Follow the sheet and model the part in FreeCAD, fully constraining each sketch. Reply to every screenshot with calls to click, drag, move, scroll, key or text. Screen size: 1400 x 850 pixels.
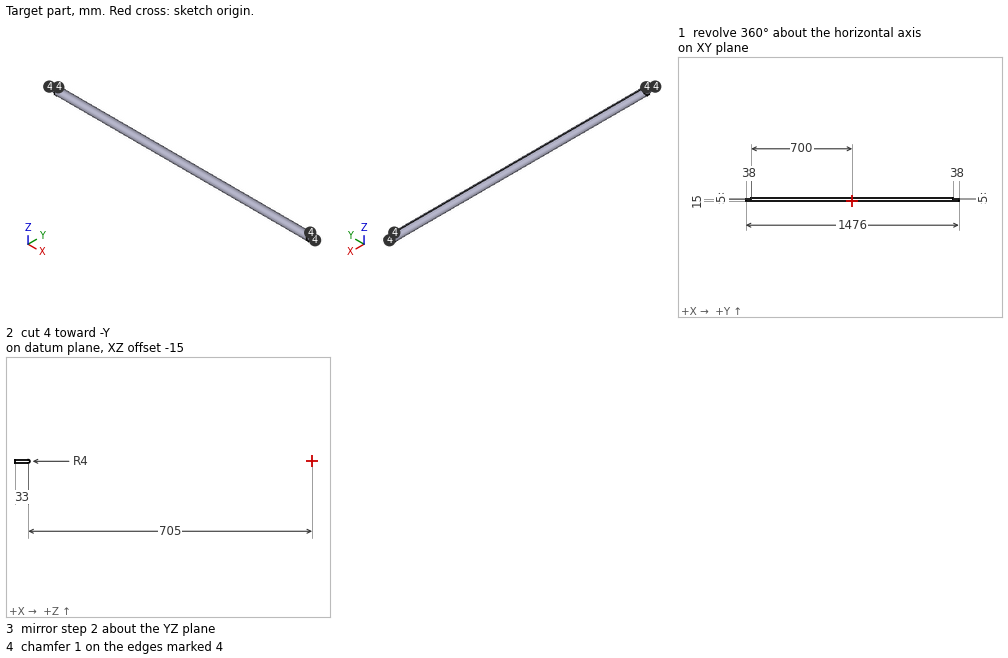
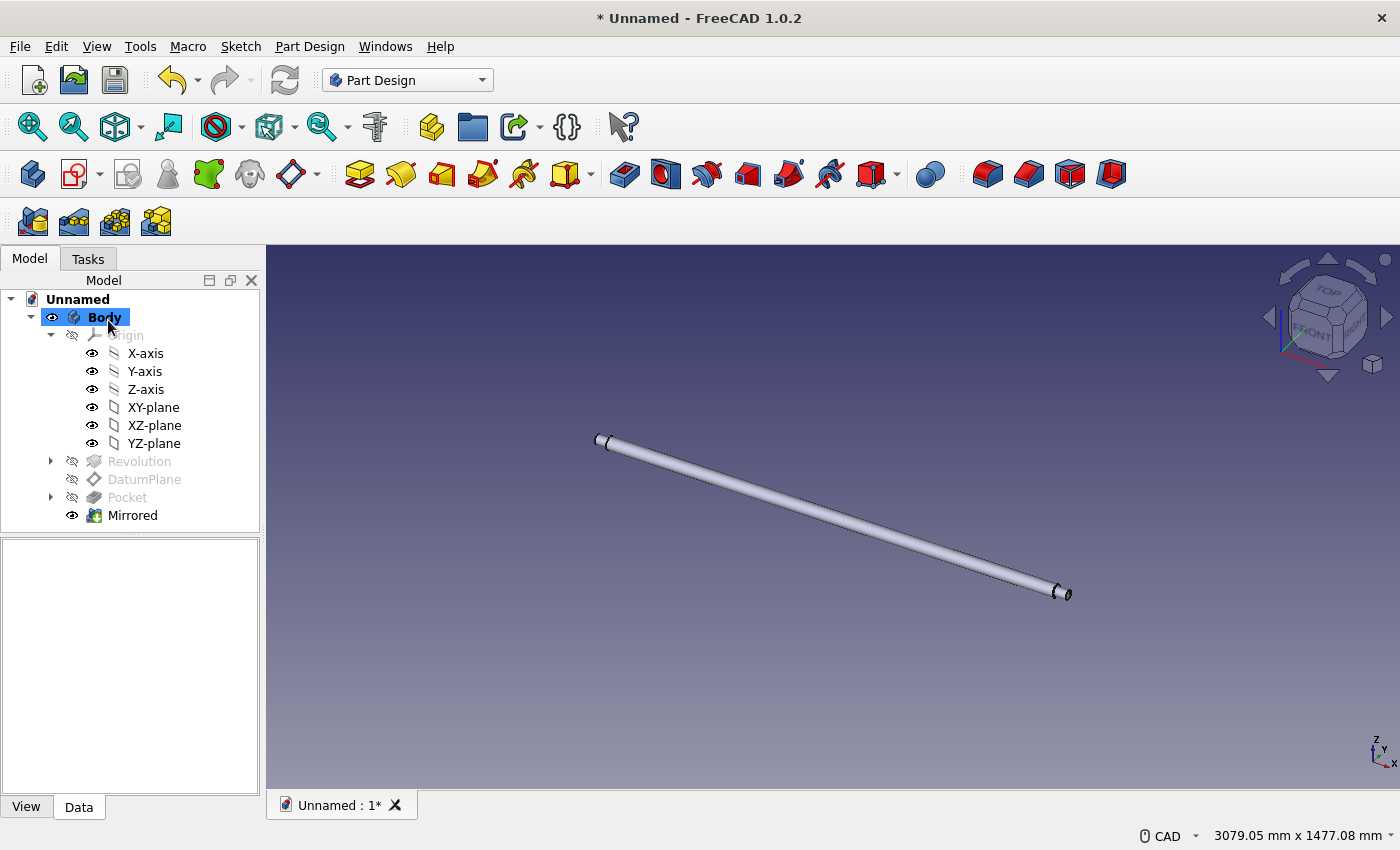
click(33, 128)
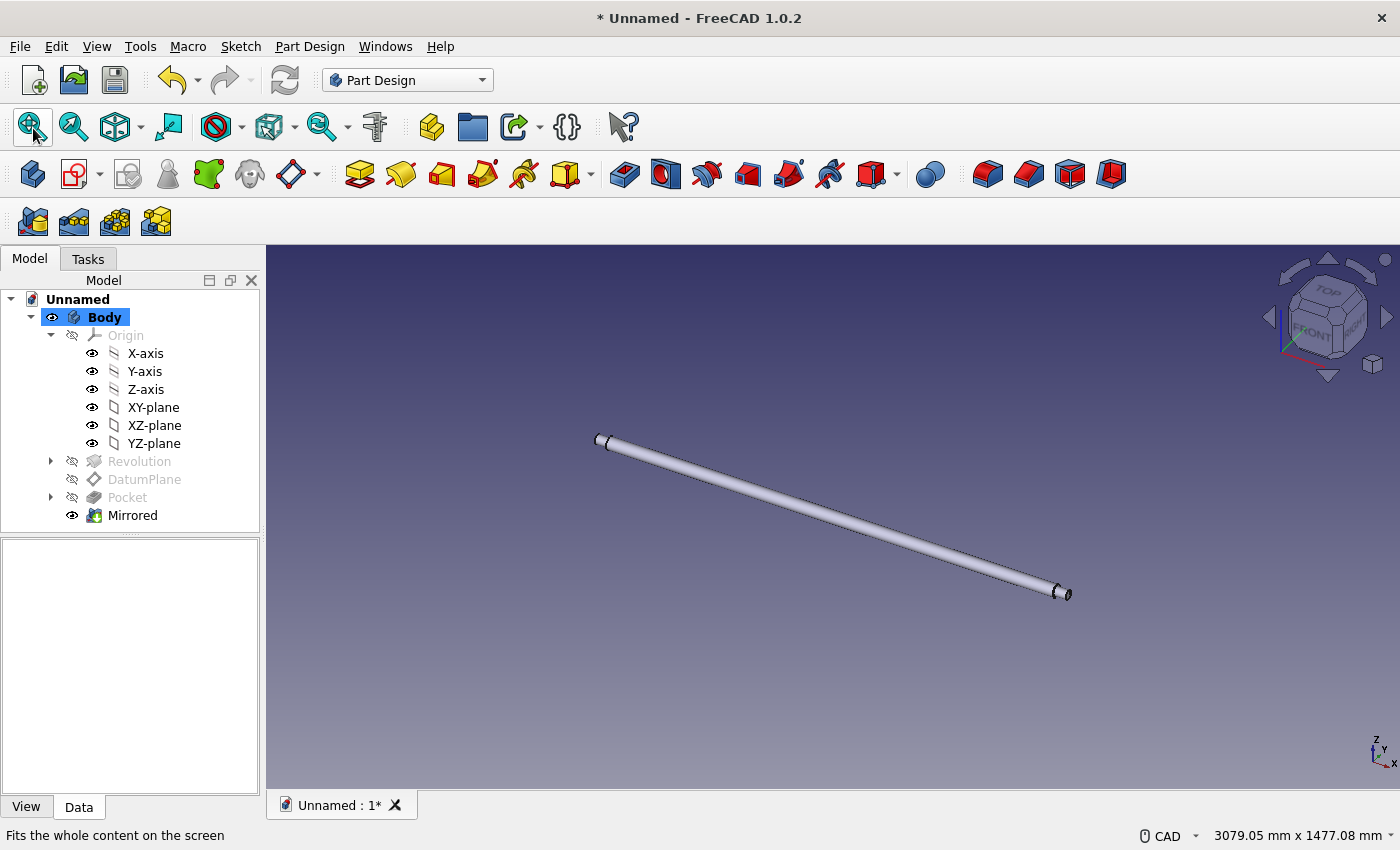
click(595, 441)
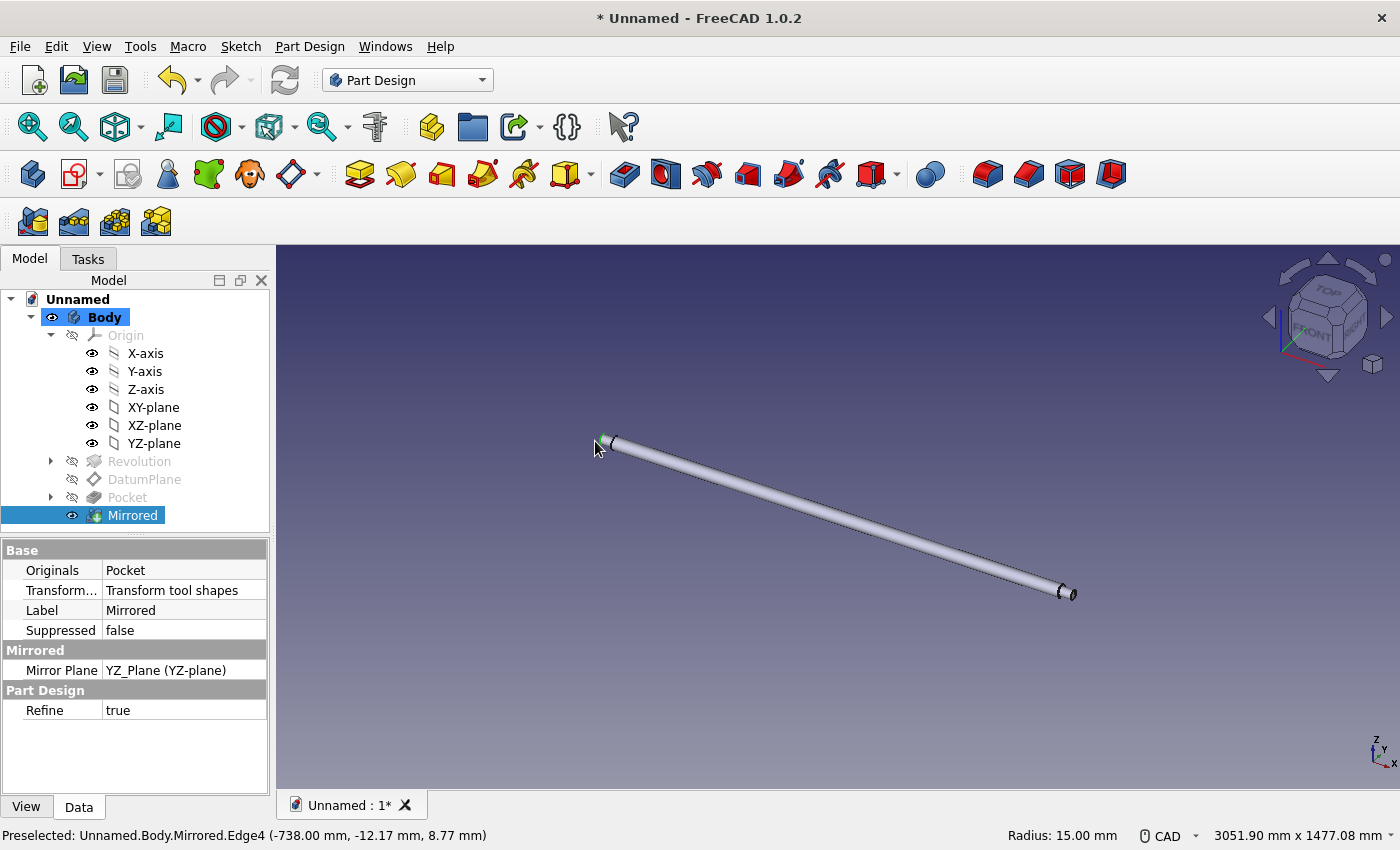
click(1071, 597, ctrl)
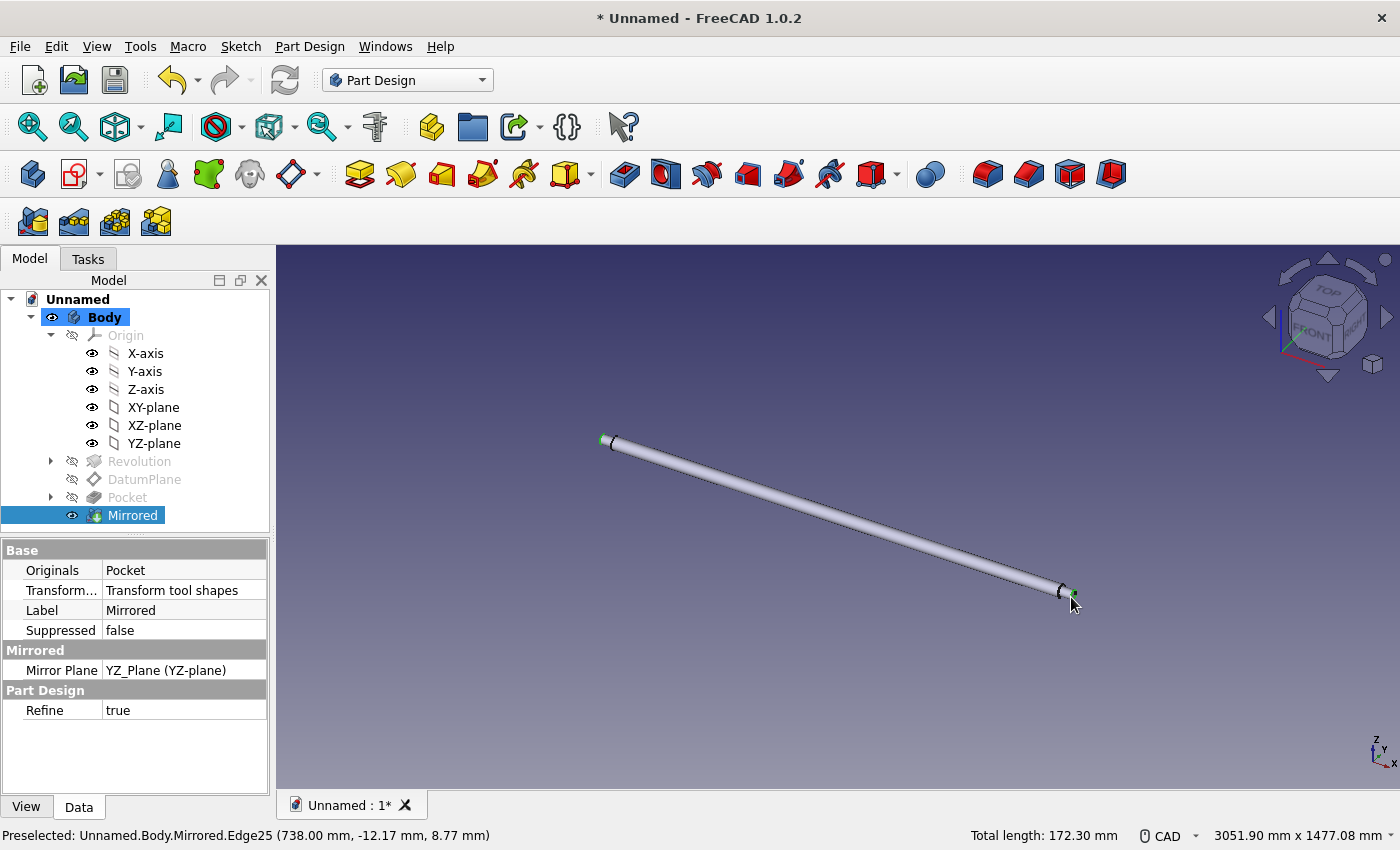
click(1058, 594, ctrl)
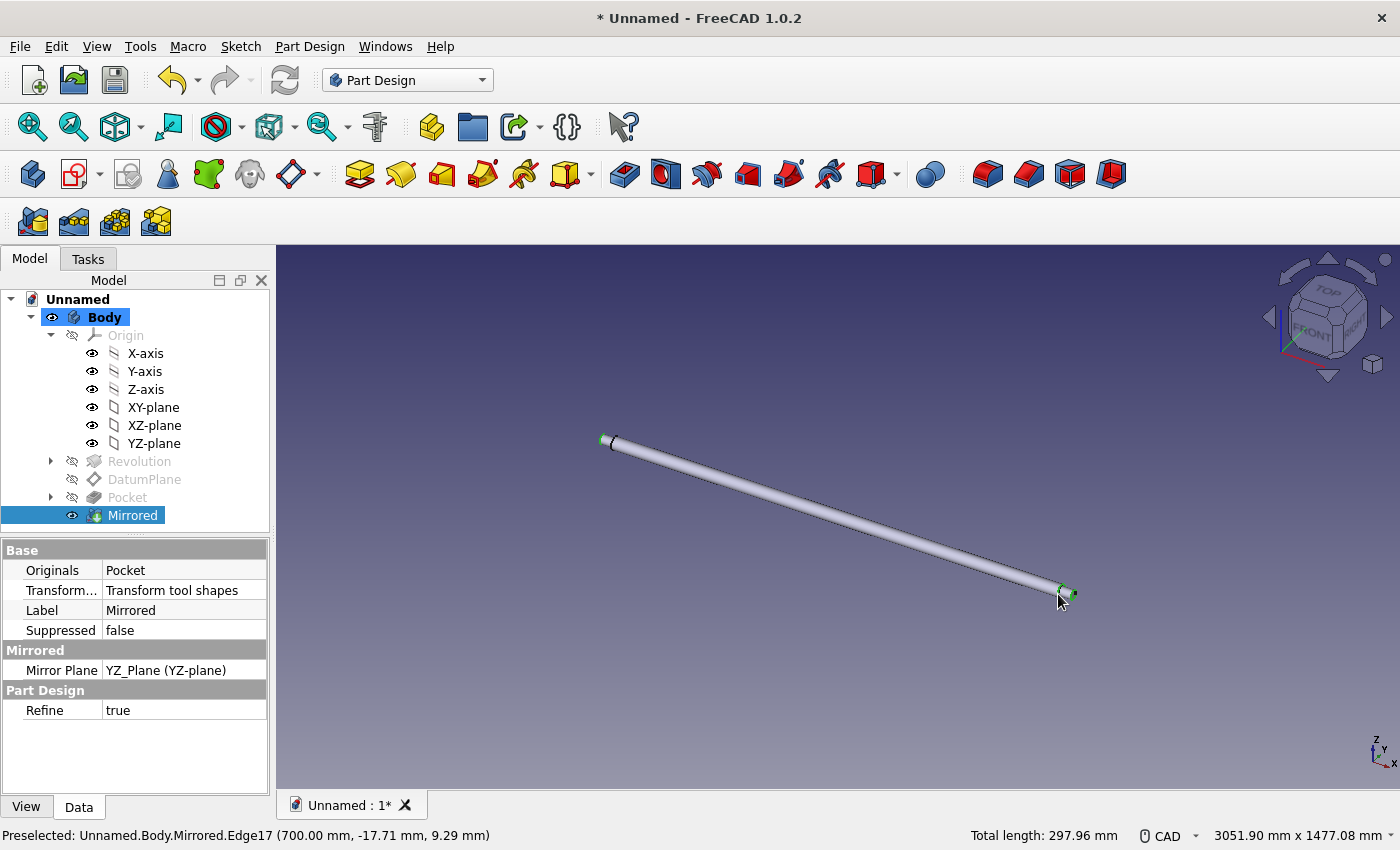
click(611, 446, ctrl)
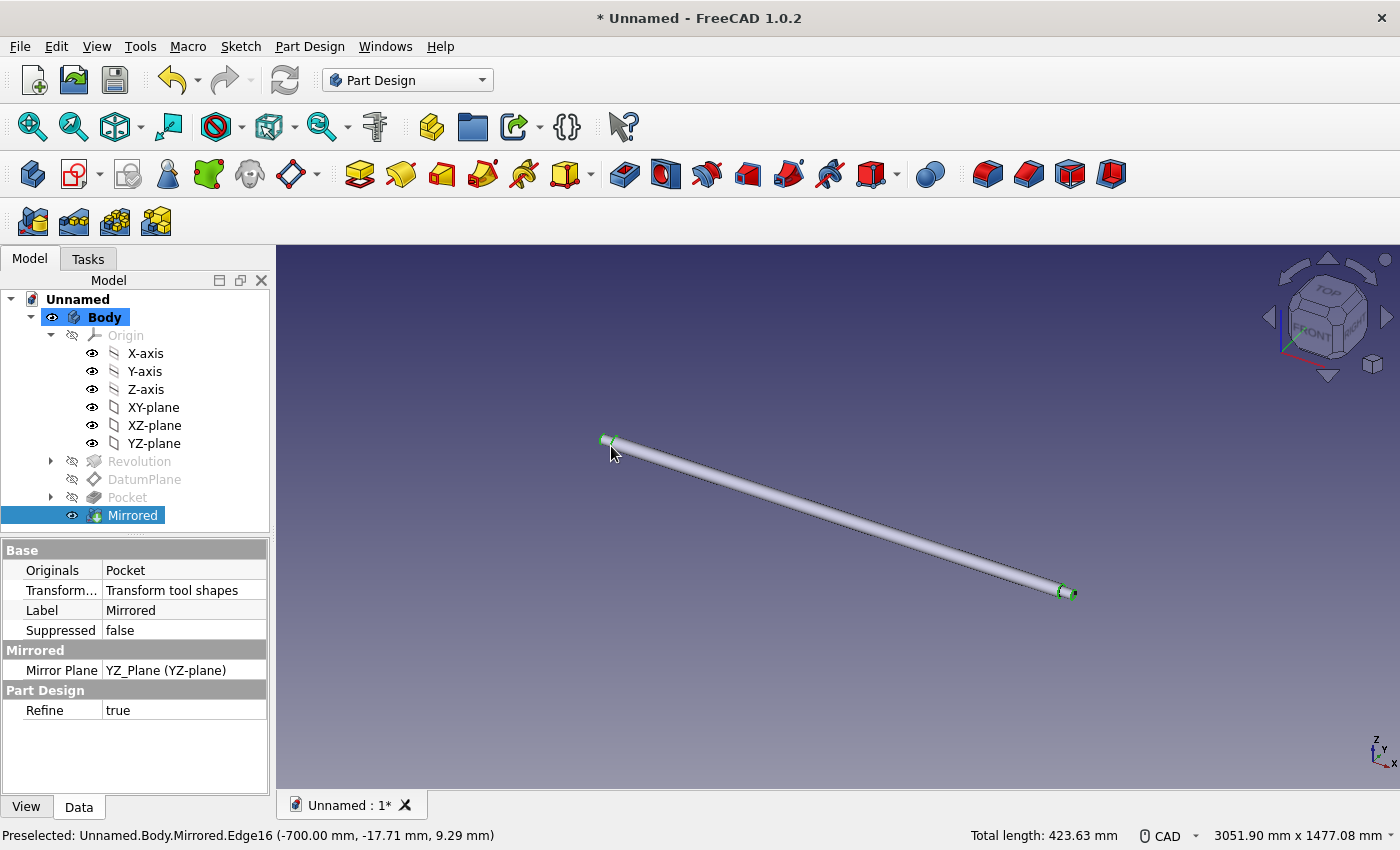
click(1029, 174)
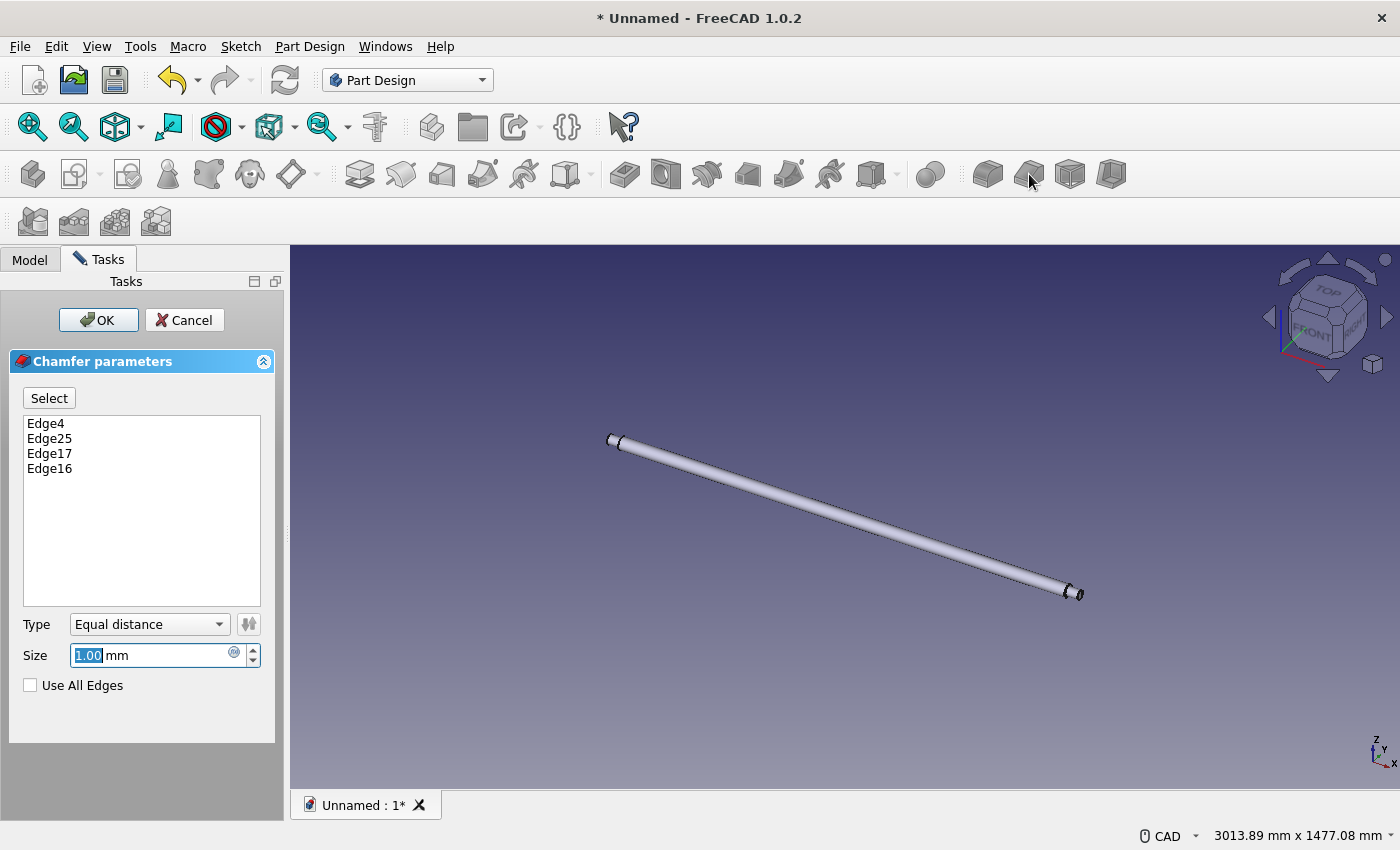
text(1)
key(Tab)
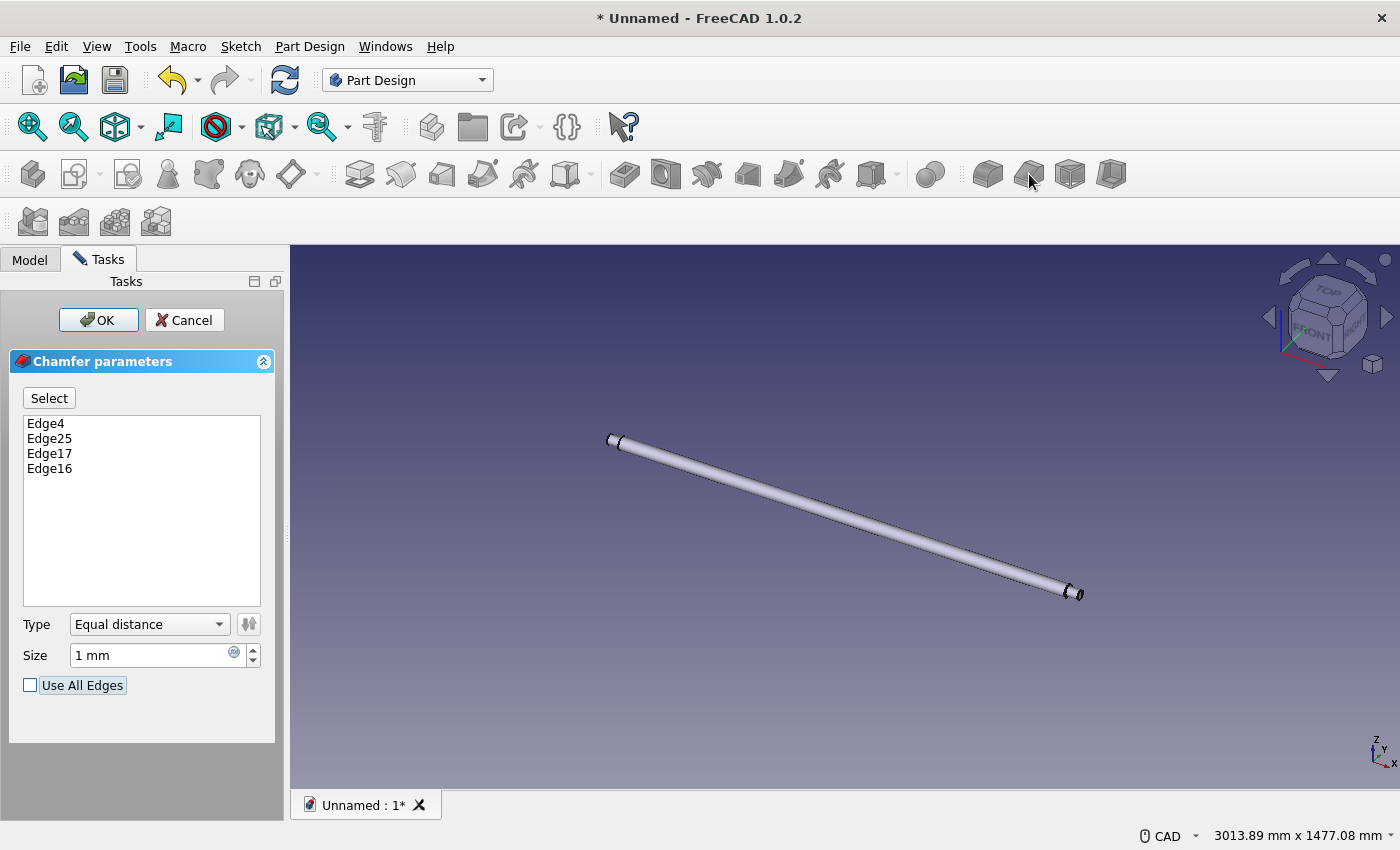
click(99, 320)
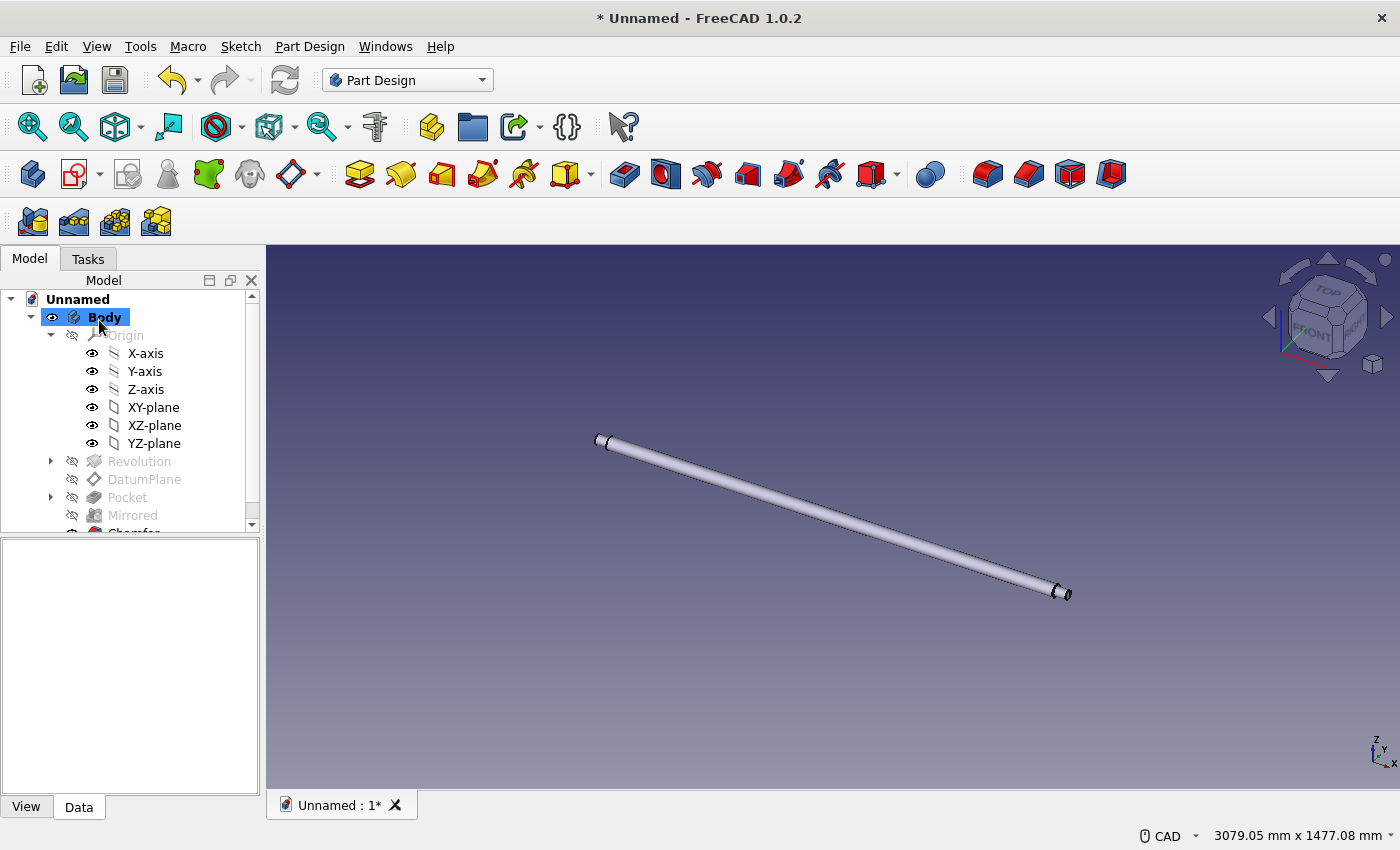
key(0)